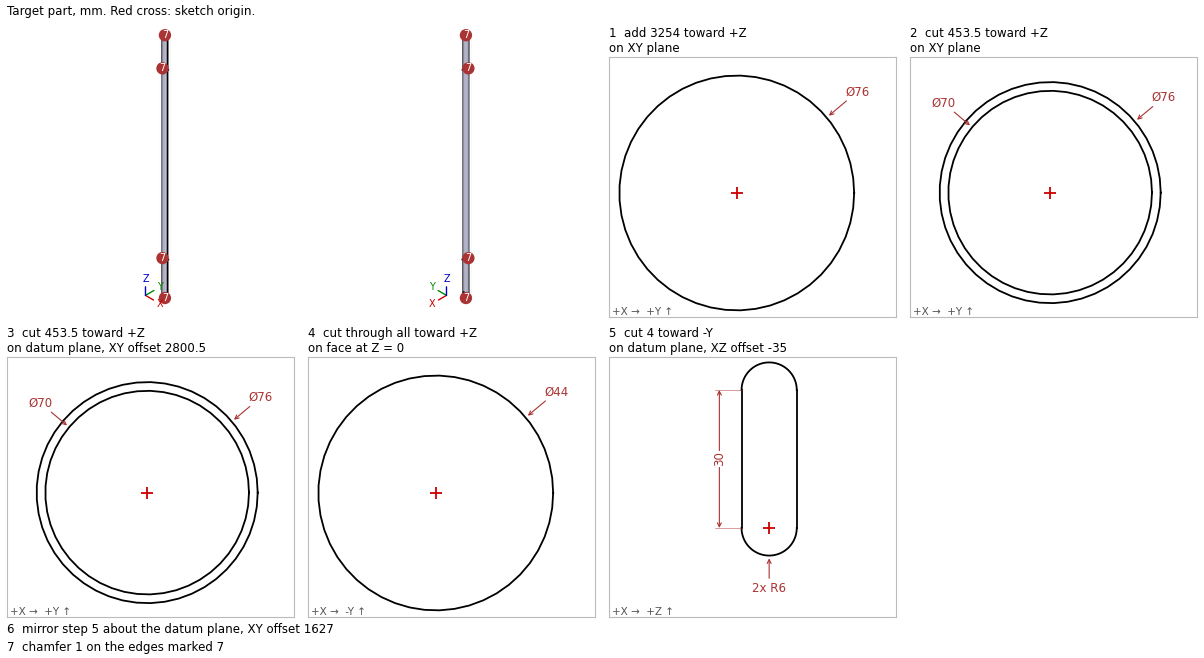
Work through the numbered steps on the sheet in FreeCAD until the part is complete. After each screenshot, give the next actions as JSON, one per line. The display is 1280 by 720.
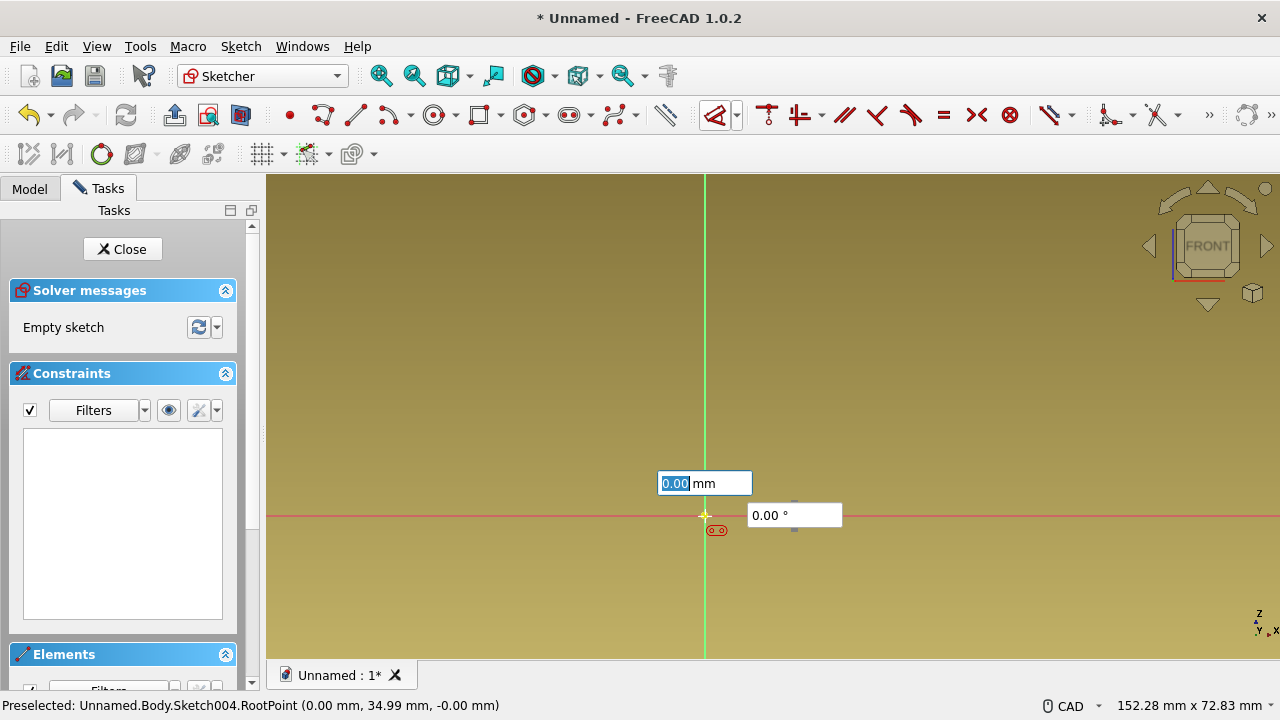
{"action": "left_click", "coordinate": [714, 316]}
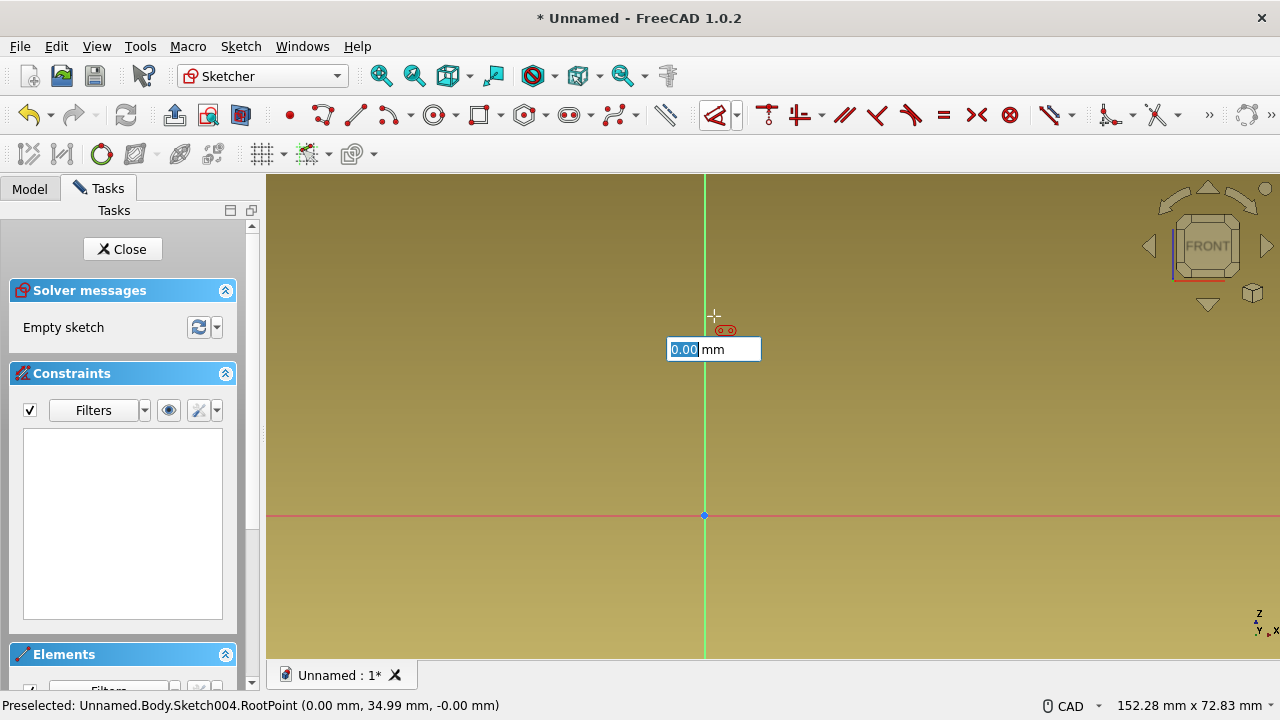
{"action": "left_click", "coordinate": [745, 416]}
{"action": "key", "text": "Escape"}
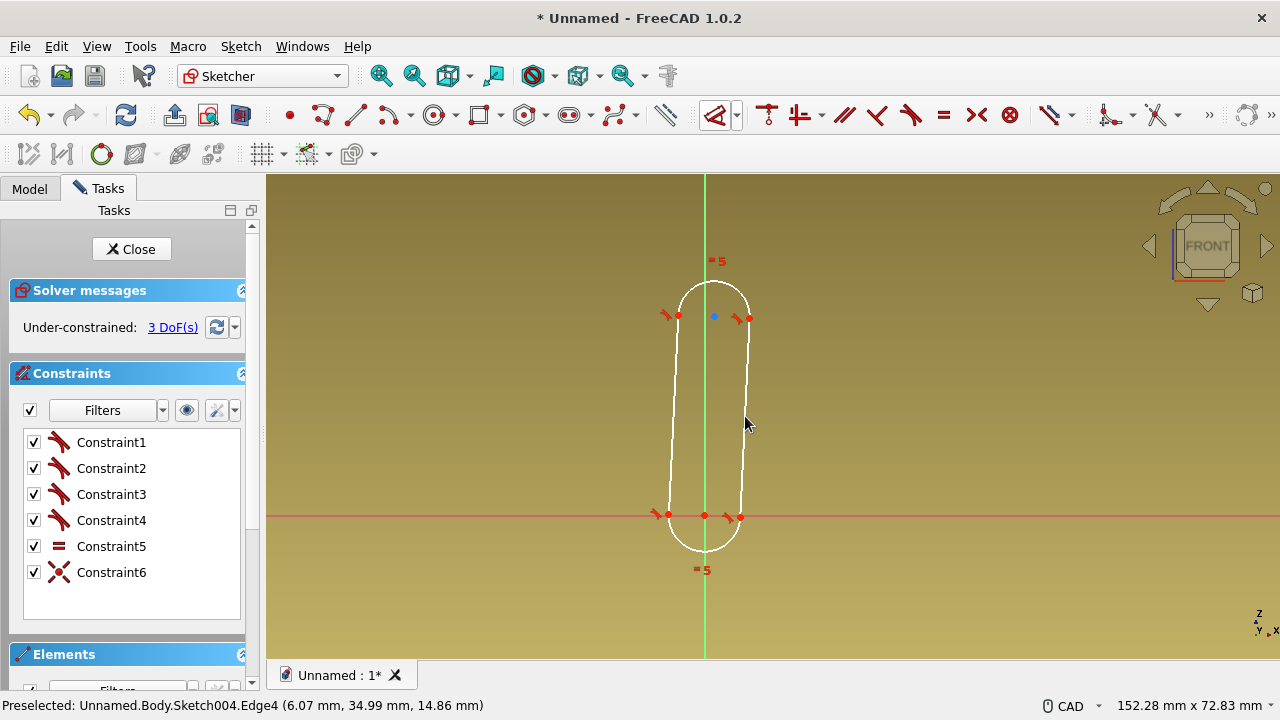
{"action": "left_click", "coordinate": [672, 455]}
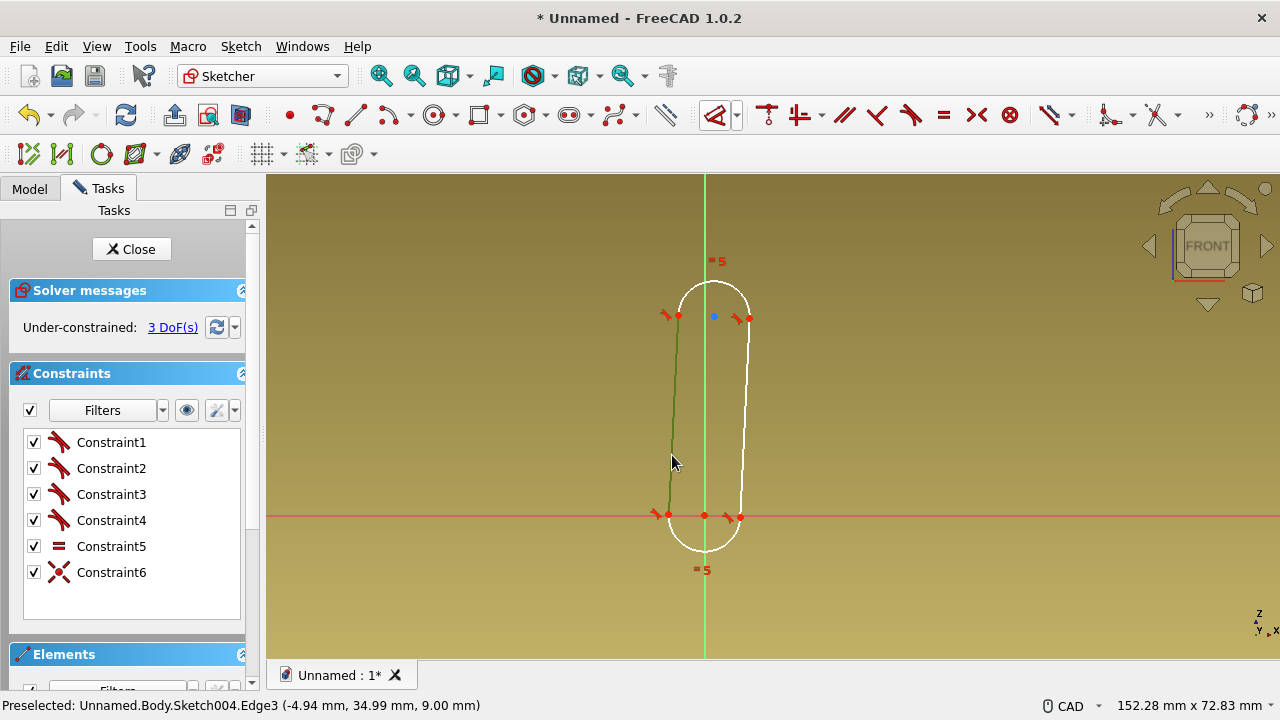
{"action": "left_click", "coordinate": [822, 116]}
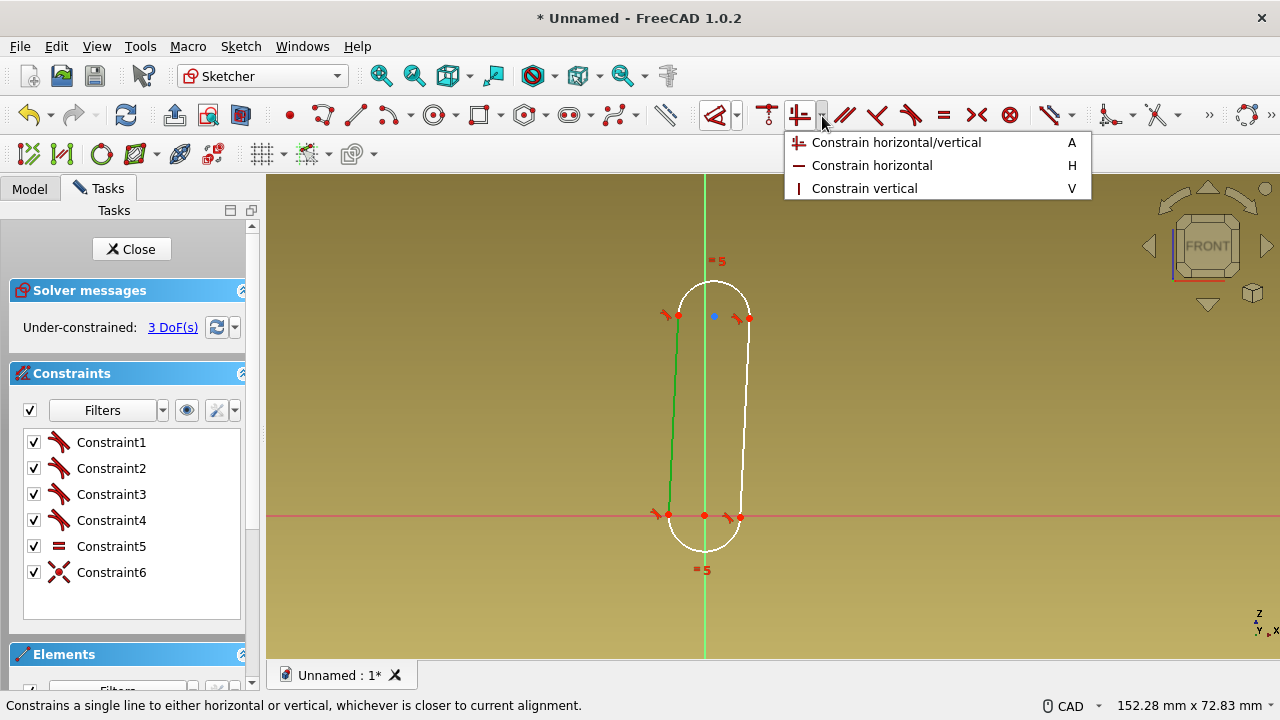
{"action": "left_click", "coordinate": [938, 188]}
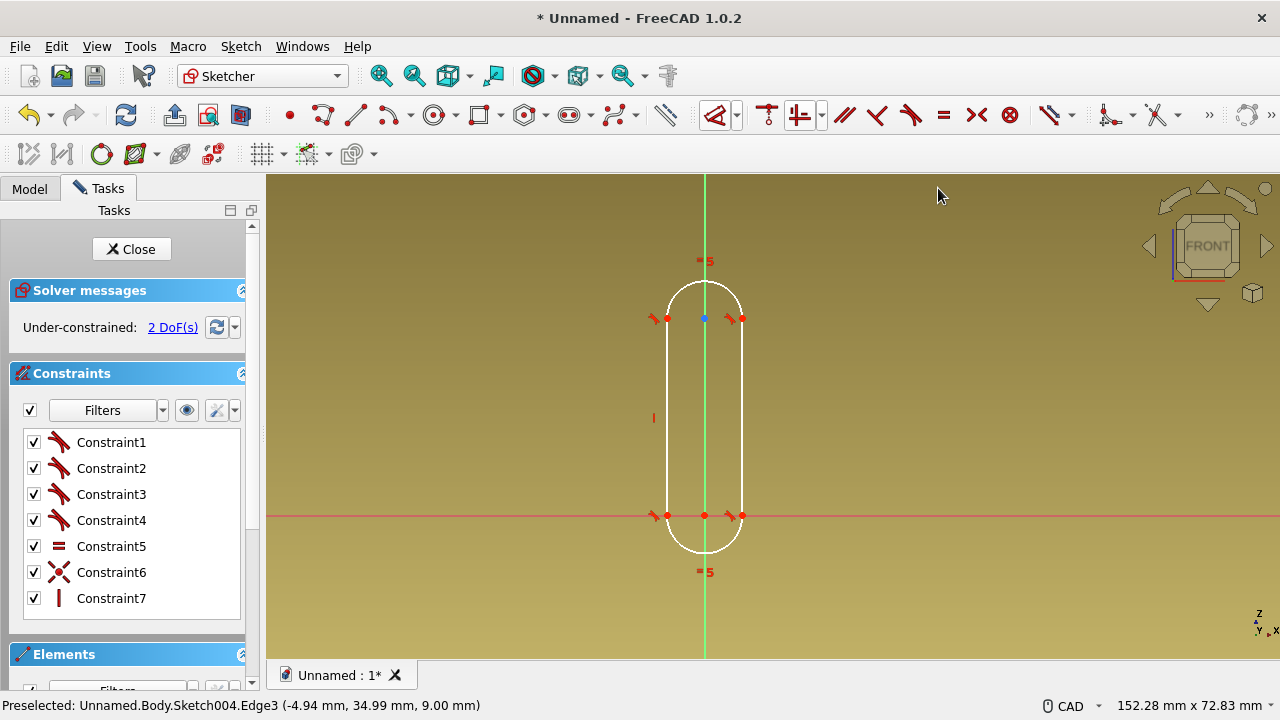
{"action": "left_click", "coordinate": [682, 546]}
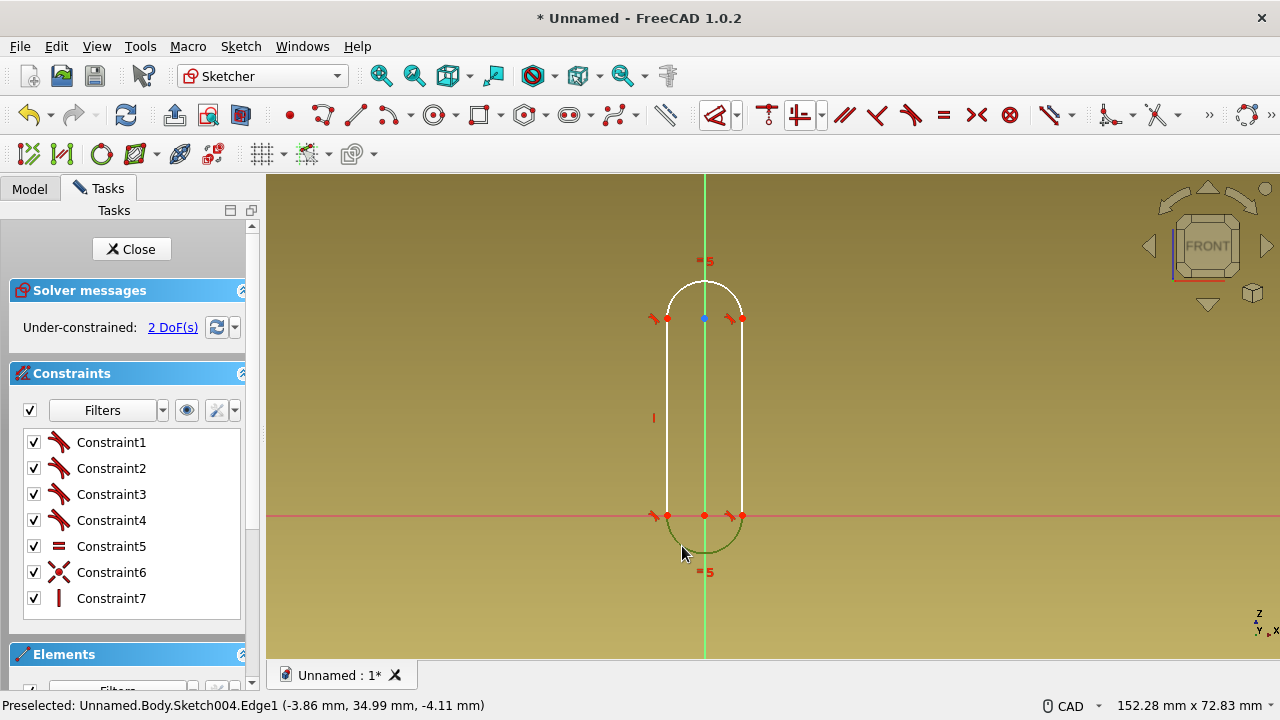
{"action": "key", "text": "k r"}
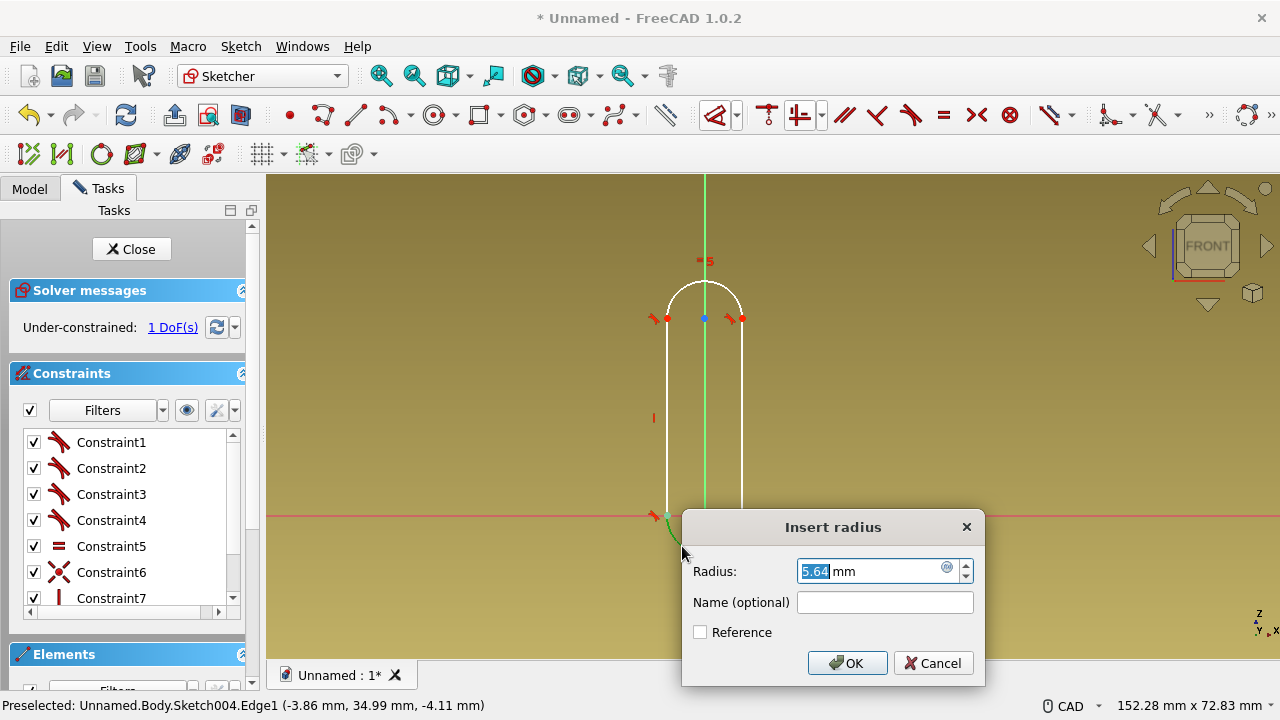
{"action": "type", "text": "6"}
{"action": "key", "text": "Return"}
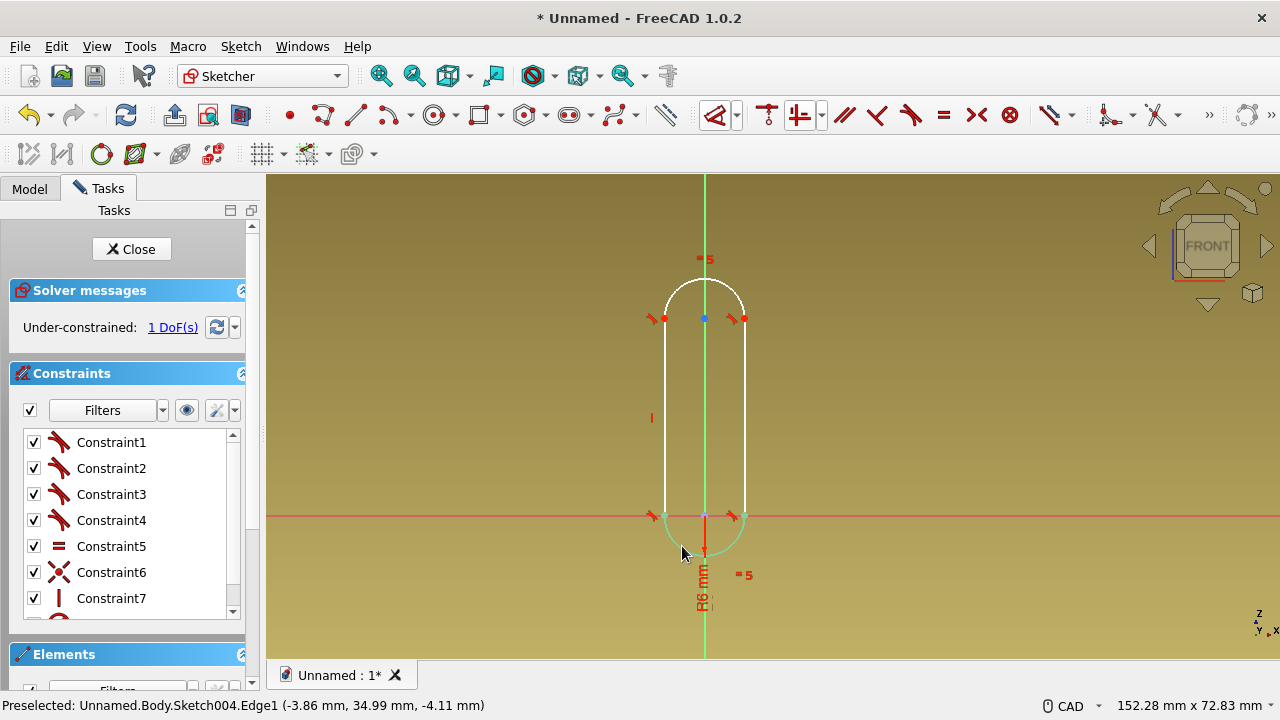
{"action": "left_click", "coordinate": [665, 457]}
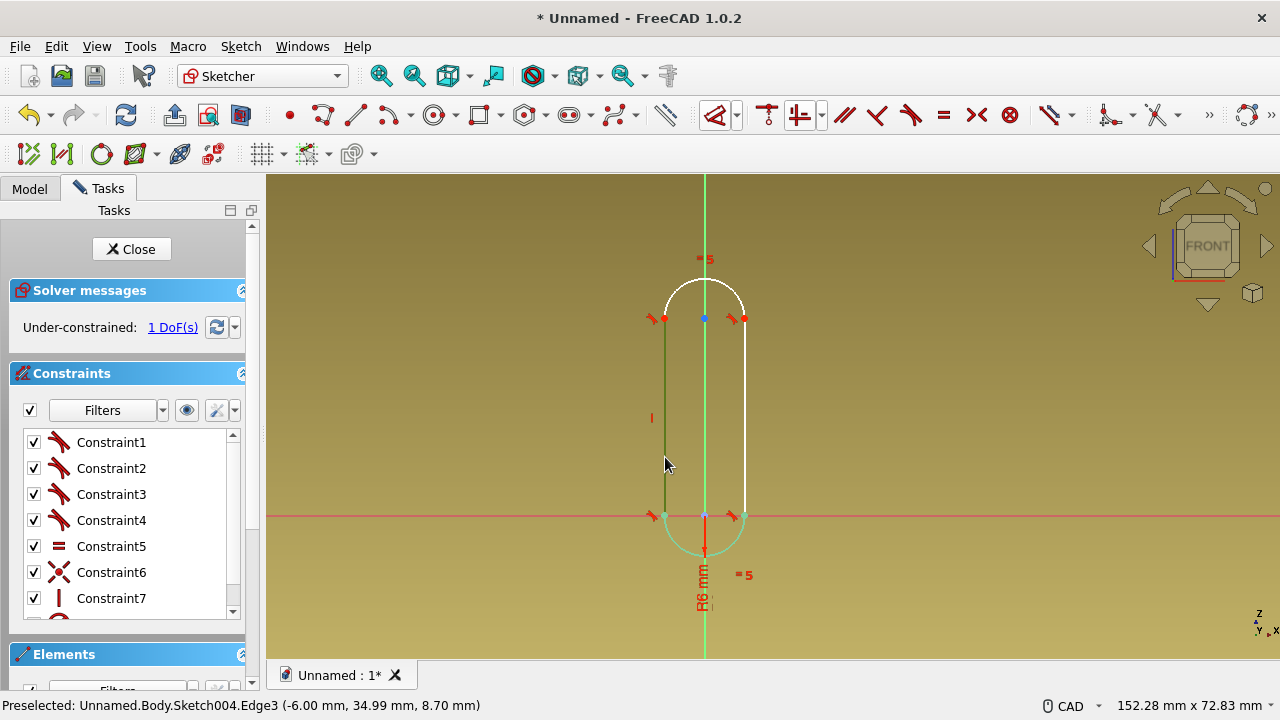
{"action": "left_click", "coordinate": [736, 116]}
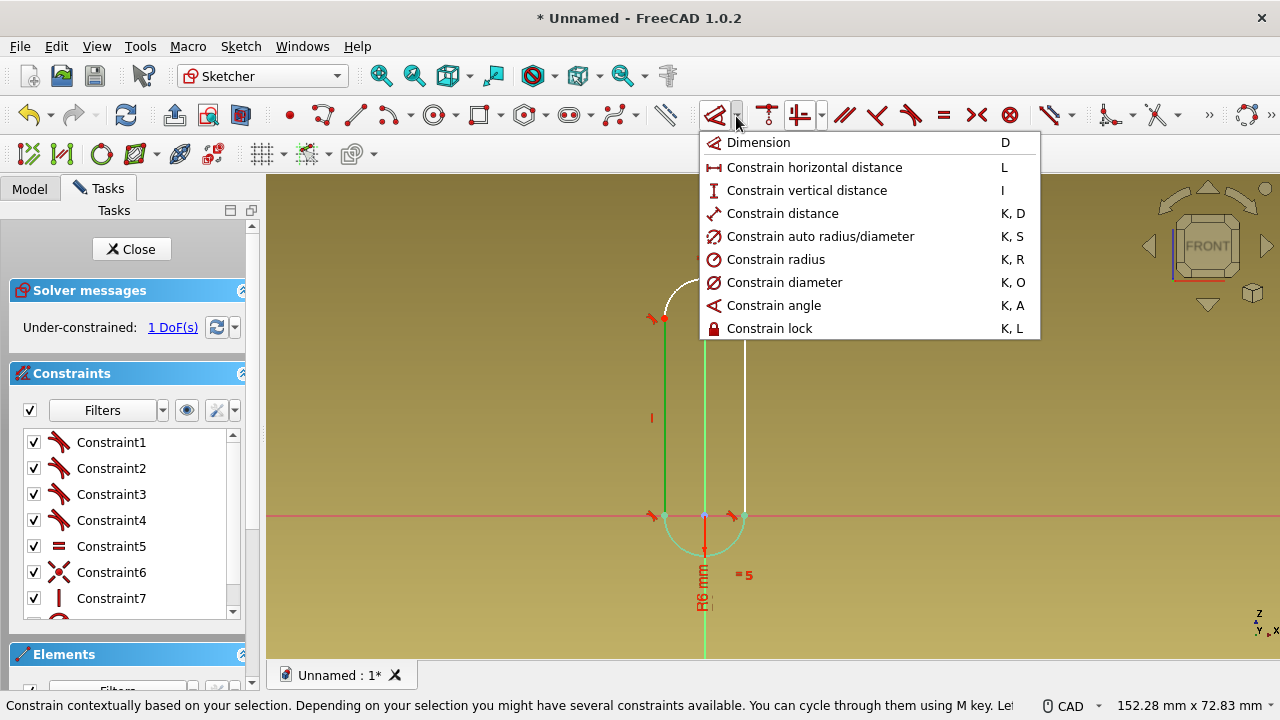
{"action": "left_click", "coordinate": [870, 190]}